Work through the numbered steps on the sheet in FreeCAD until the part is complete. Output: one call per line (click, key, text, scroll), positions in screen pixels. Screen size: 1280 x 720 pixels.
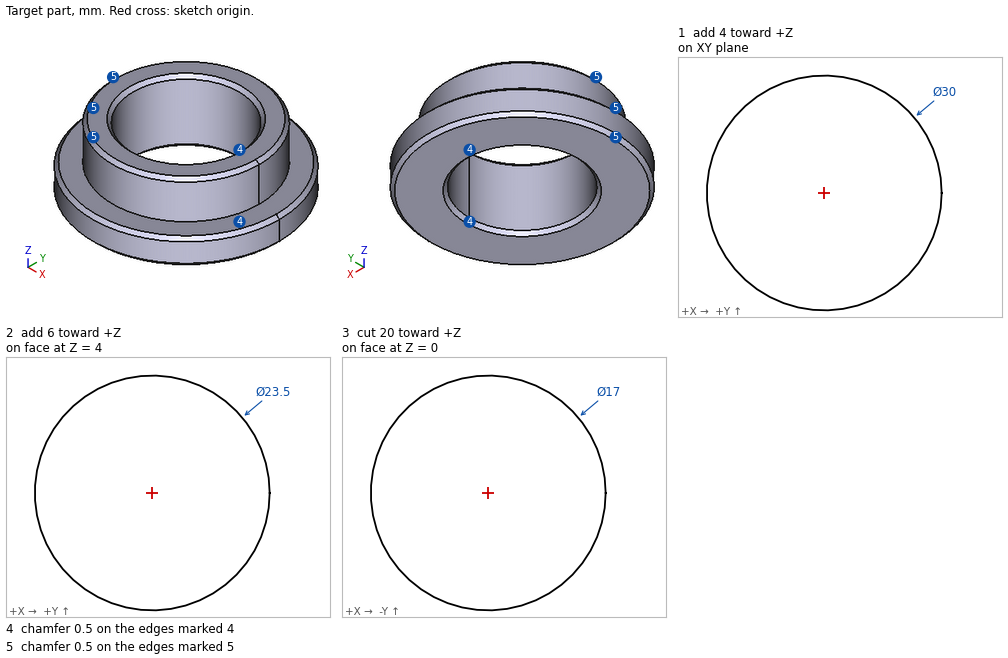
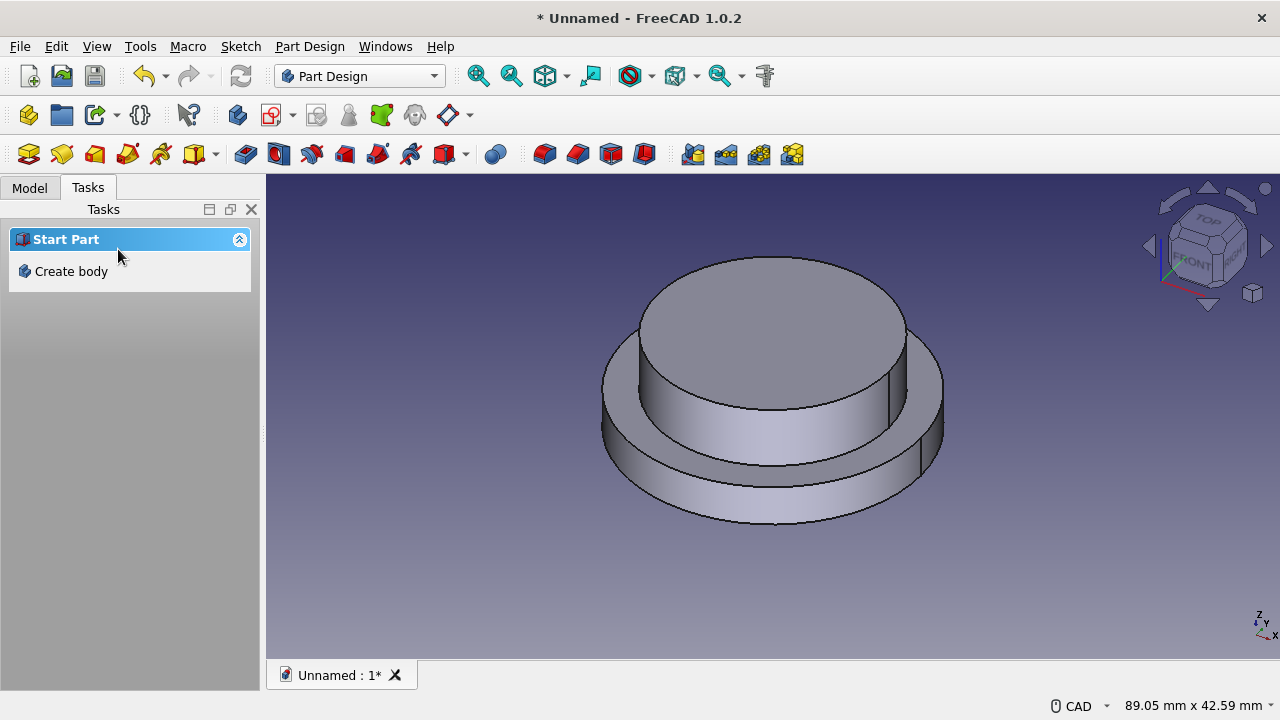
key(5)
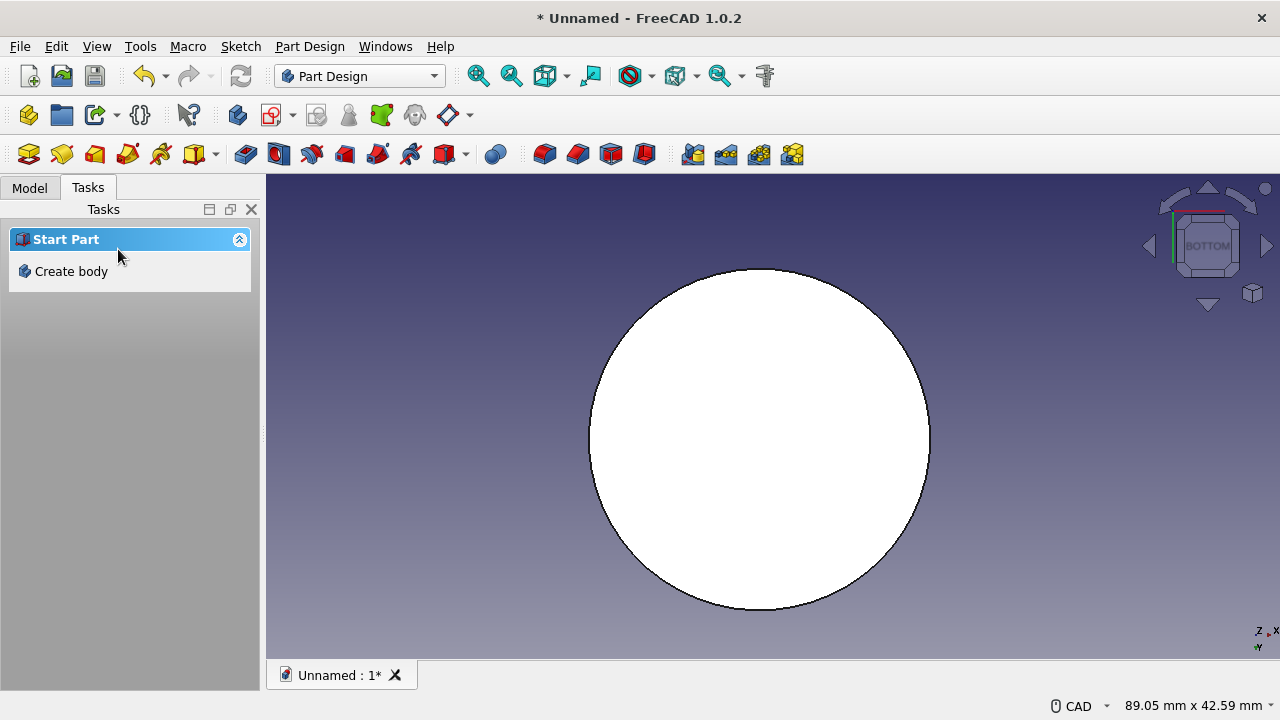
click(760, 439)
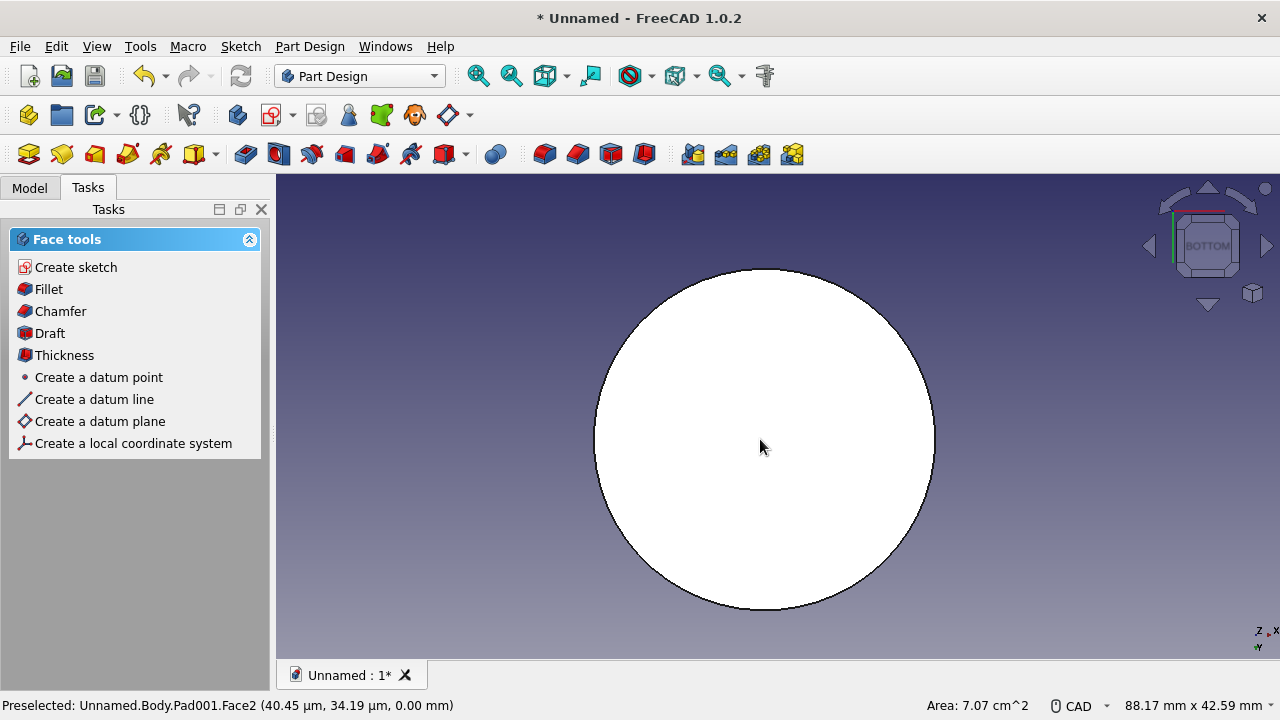
click(270, 116)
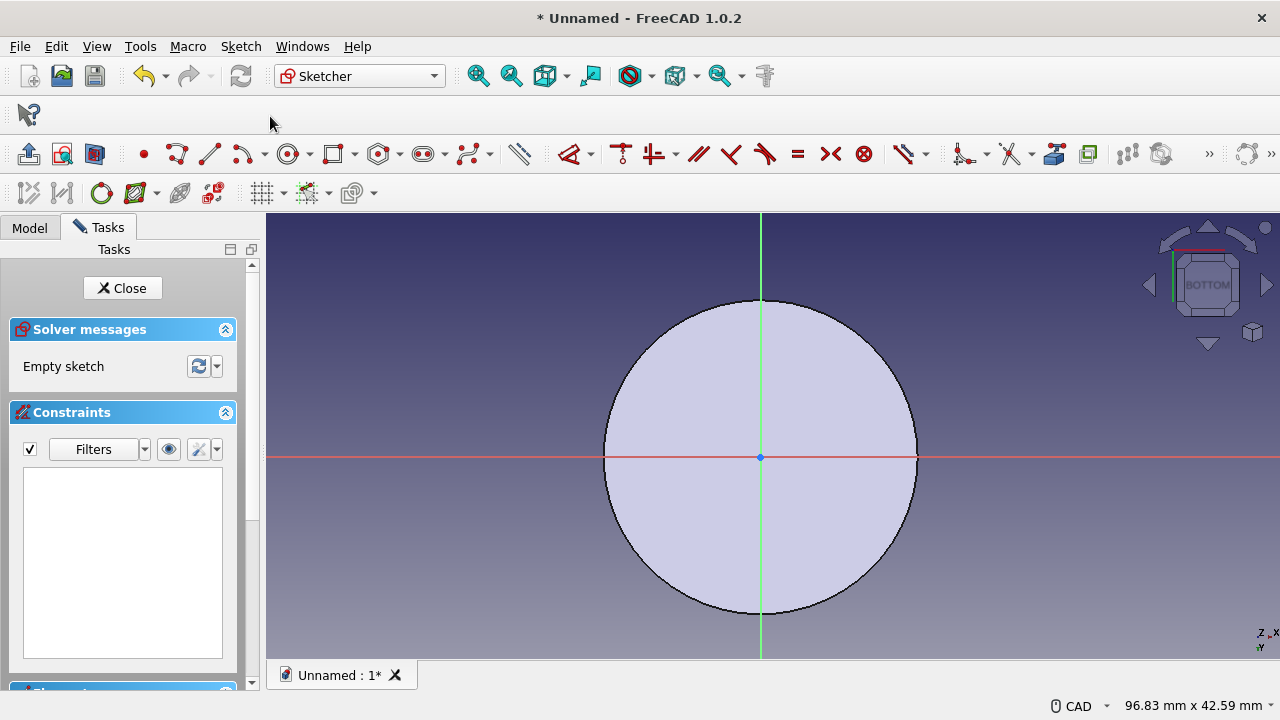
scroll(875, 500, up, 2)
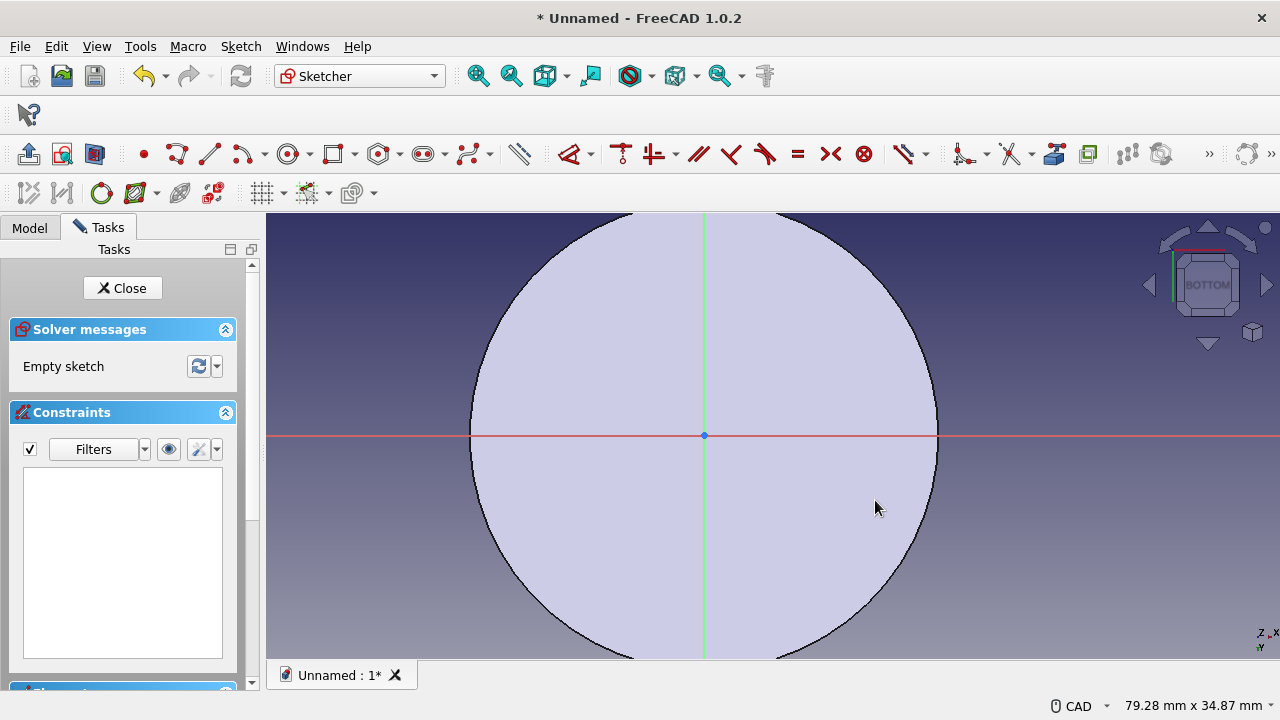
click(288, 154)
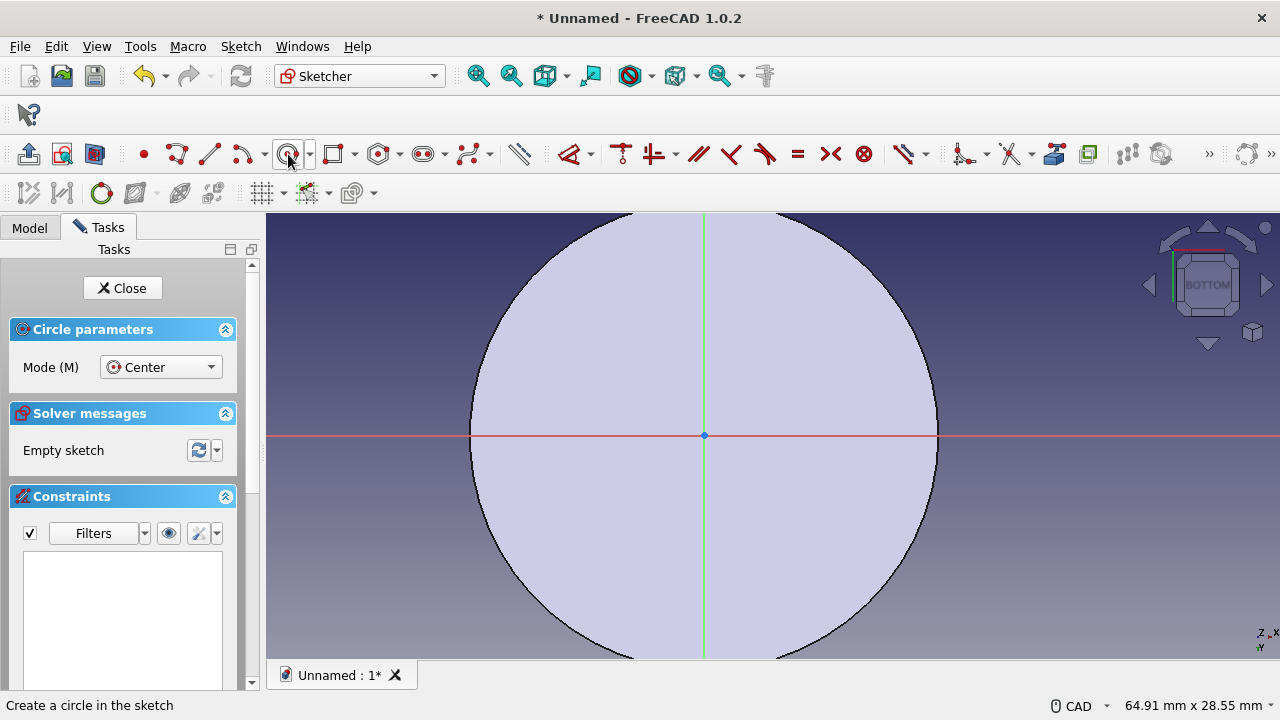
click(704, 436)
move(798, 342)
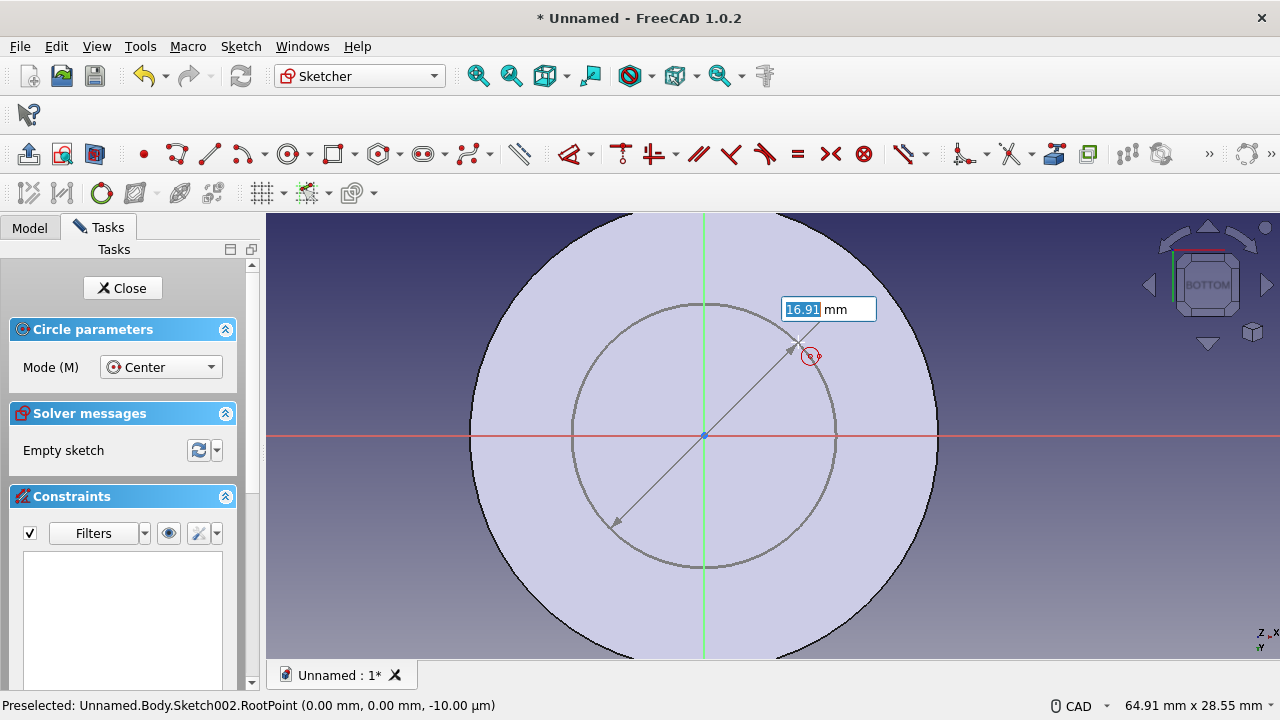
text(17)
key(Return)
key(Escape)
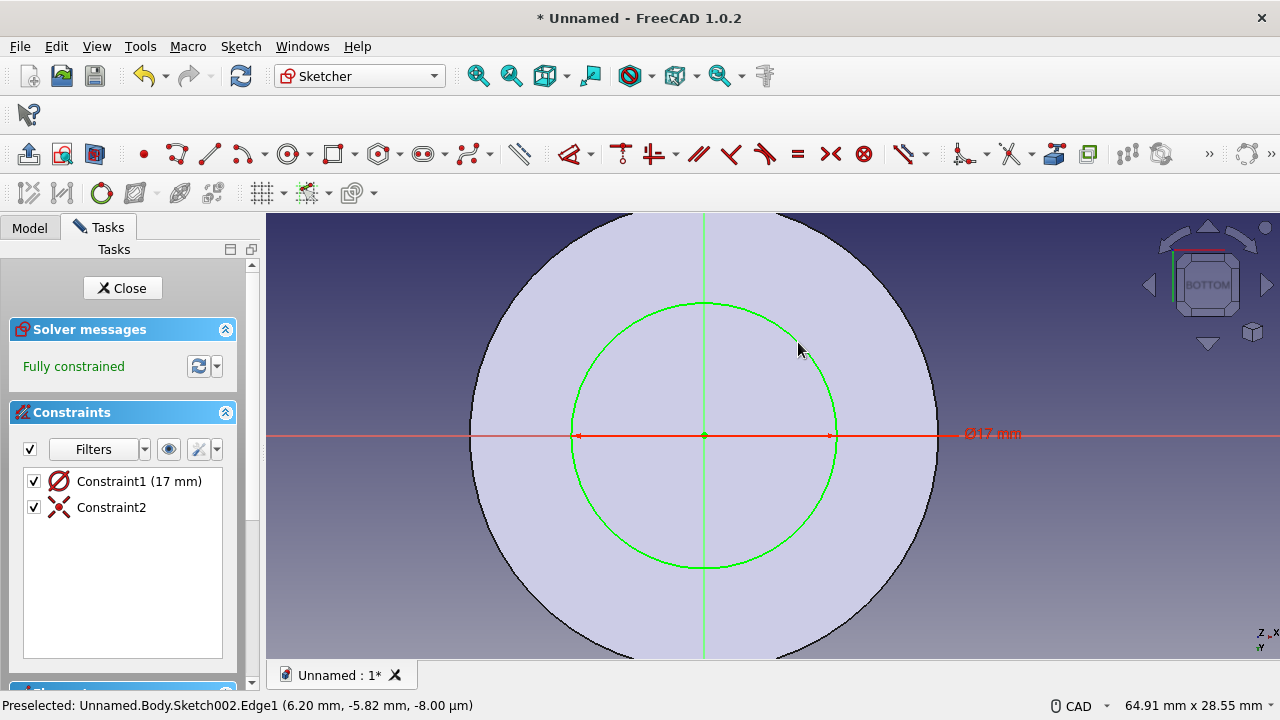
click(123, 288)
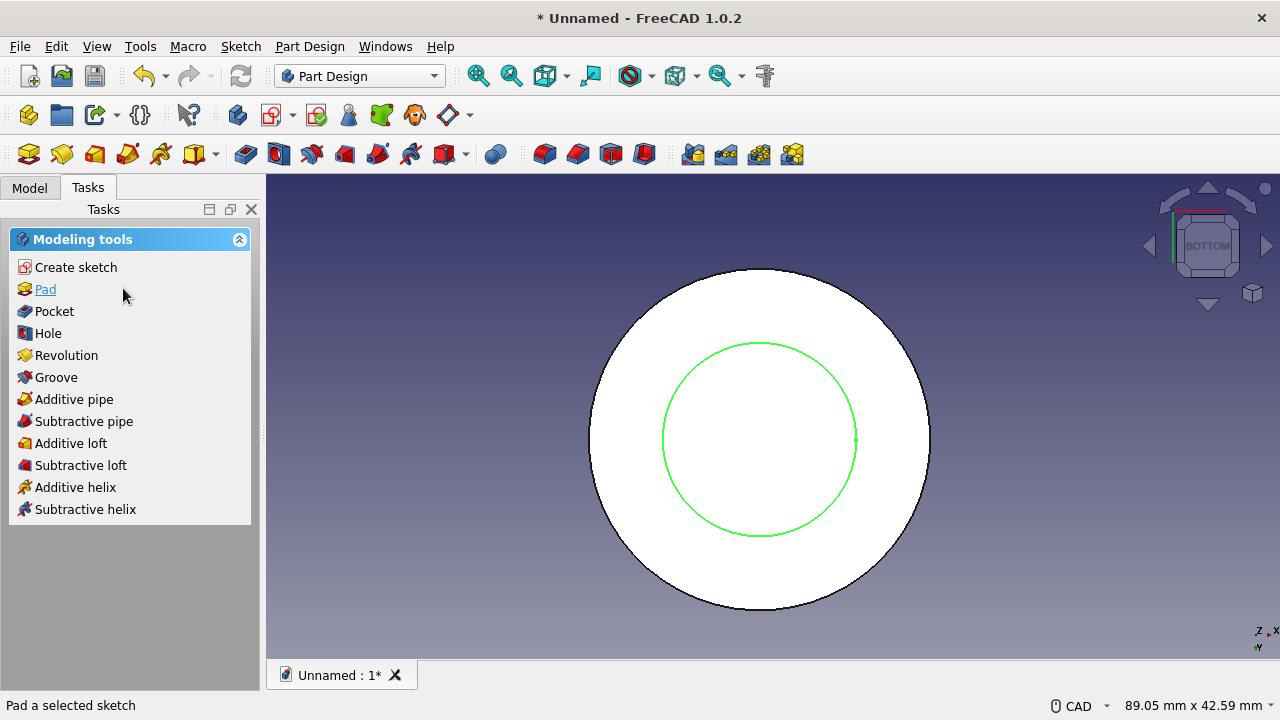
click(246, 154)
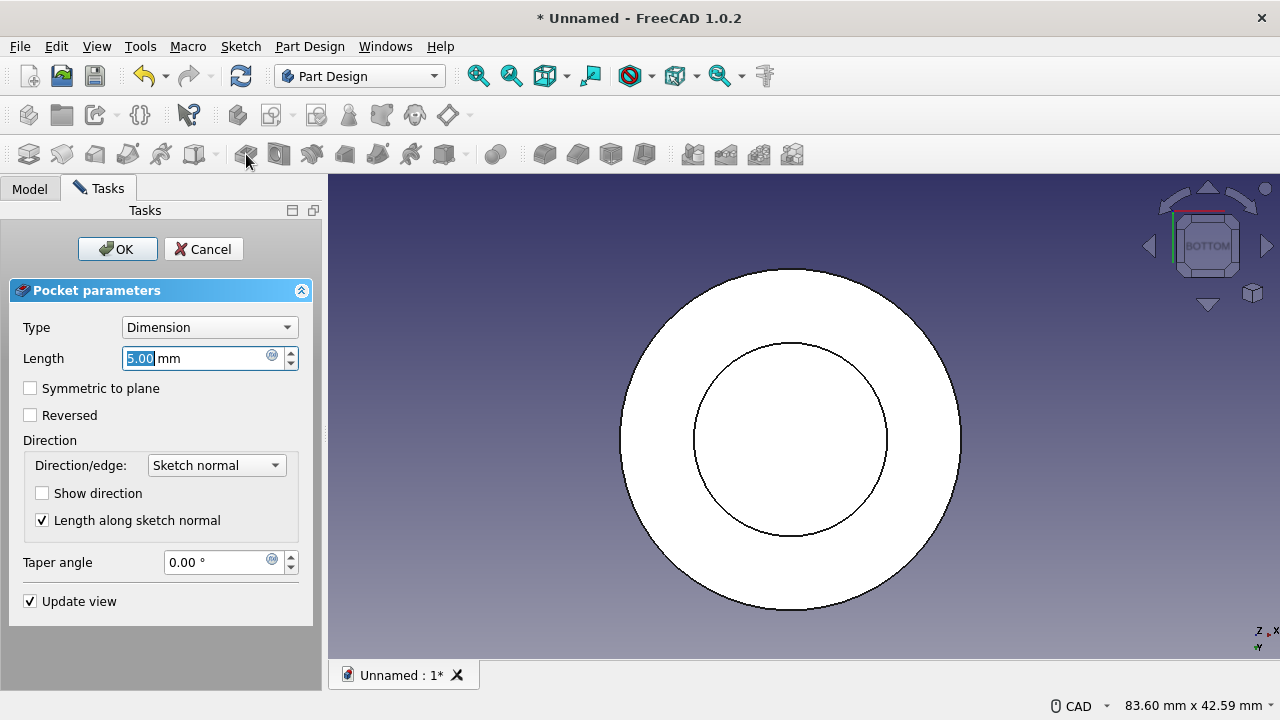
text(20)
key(Tab)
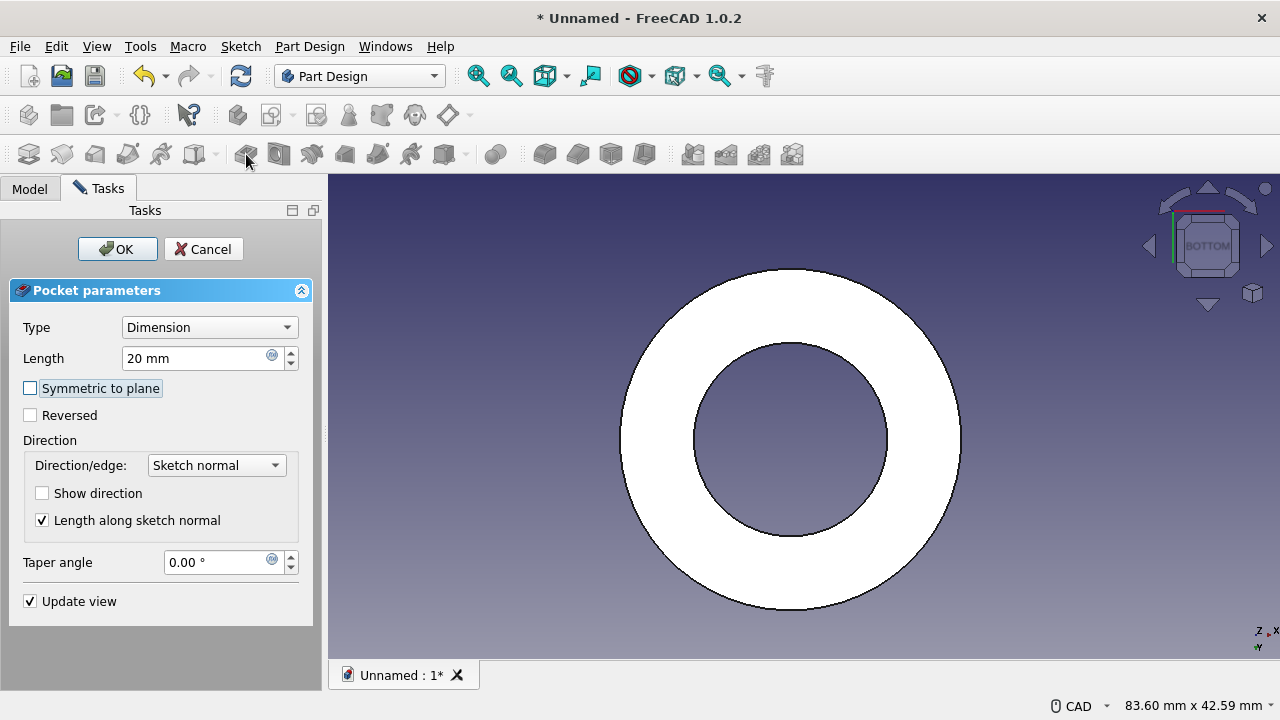
click(118, 249)